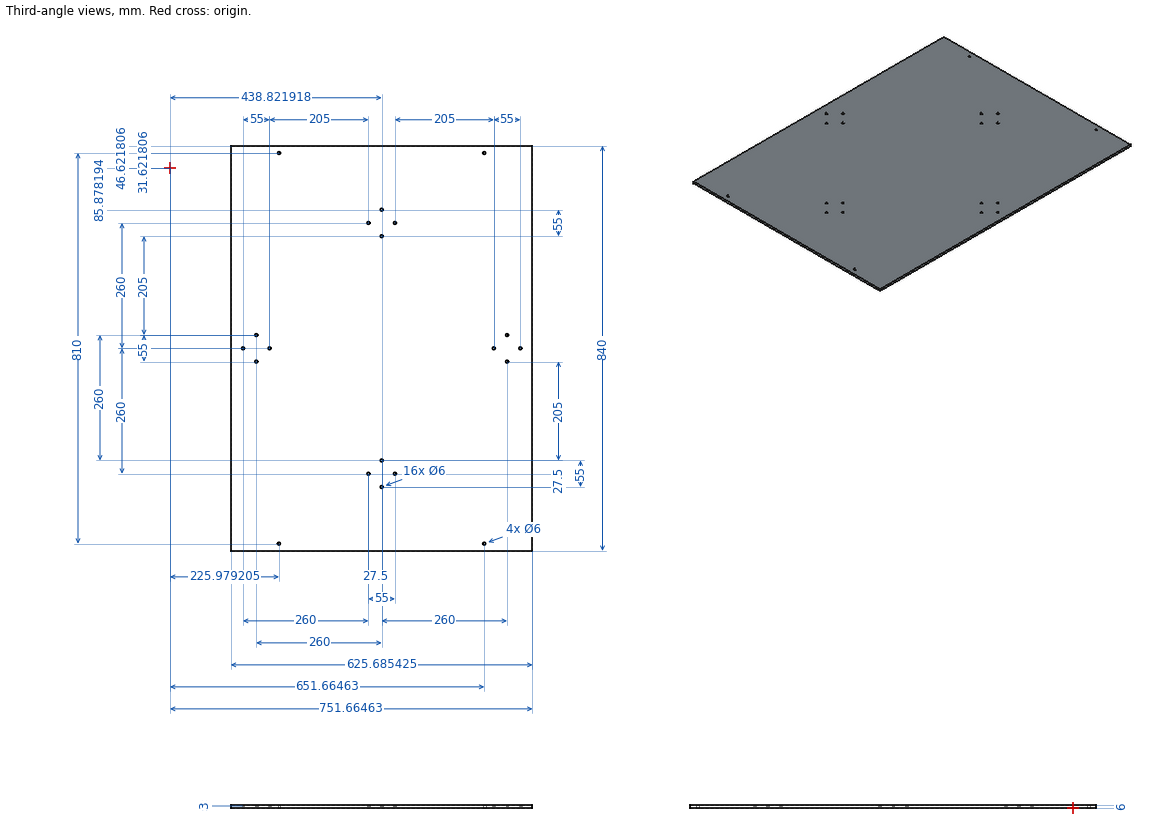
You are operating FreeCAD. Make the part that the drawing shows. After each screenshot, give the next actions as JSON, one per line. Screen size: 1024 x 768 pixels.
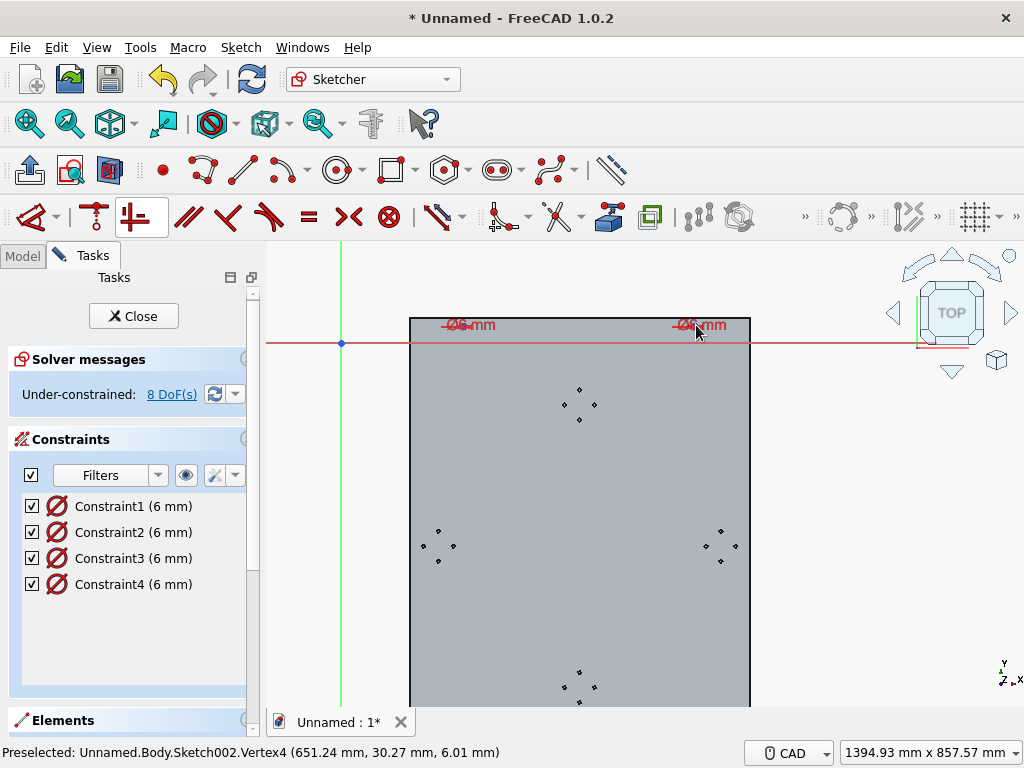
{"action": "scroll", "coordinate": [693, 327], "scroll_direction": "down", "scroll_amount": 2}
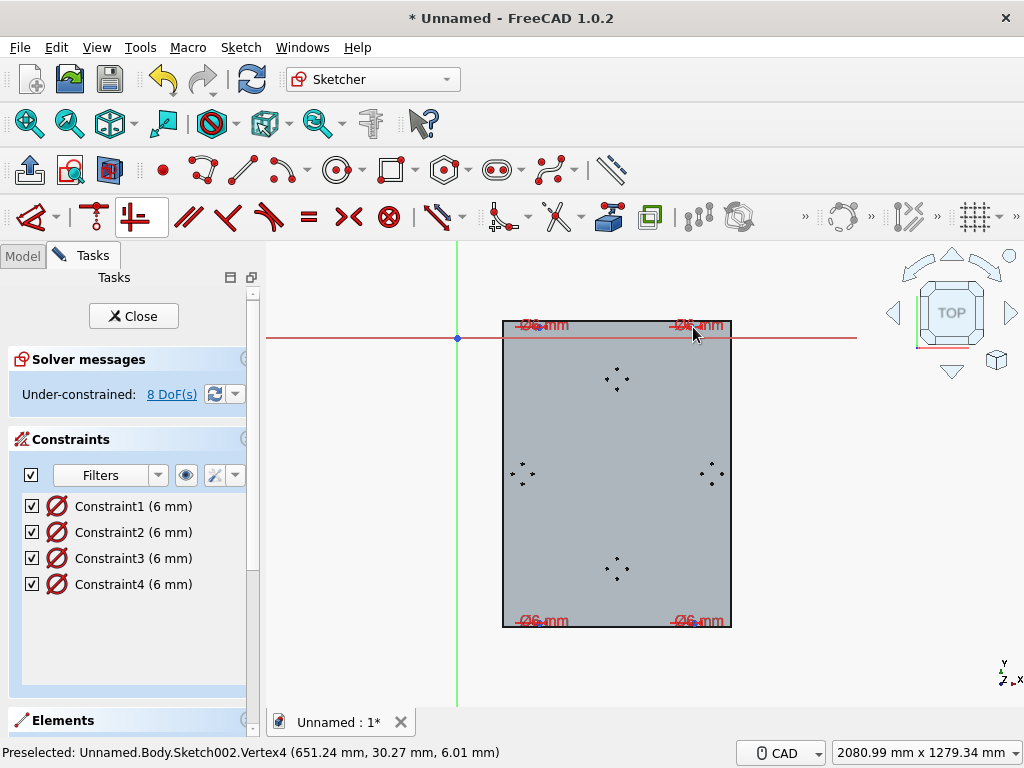
{"action": "left_click", "coordinate": [695, 623]}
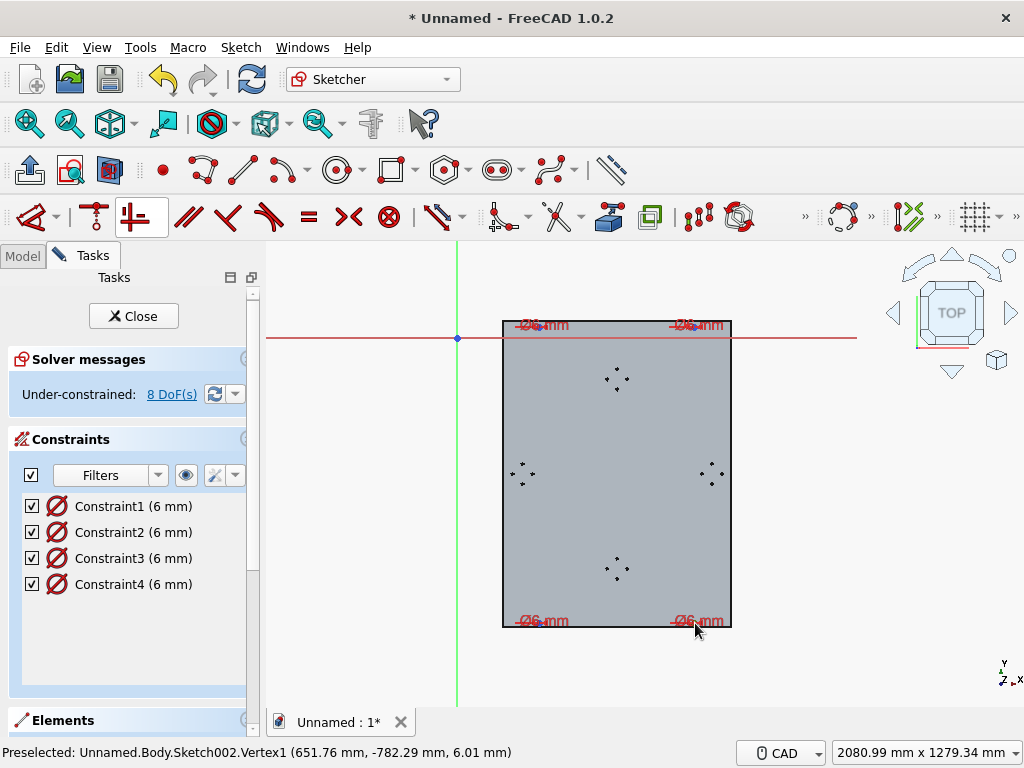
{"action": "left_click", "coordinate": [540, 623]}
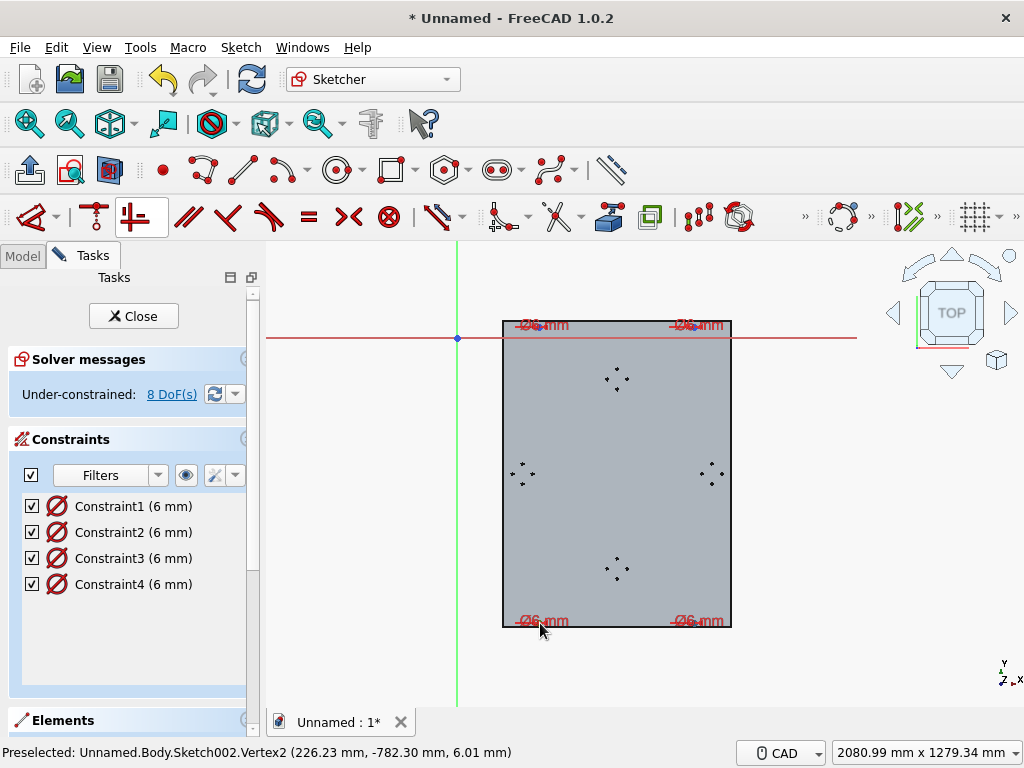
{"action": "left_click", "coordinate": [162, 218]}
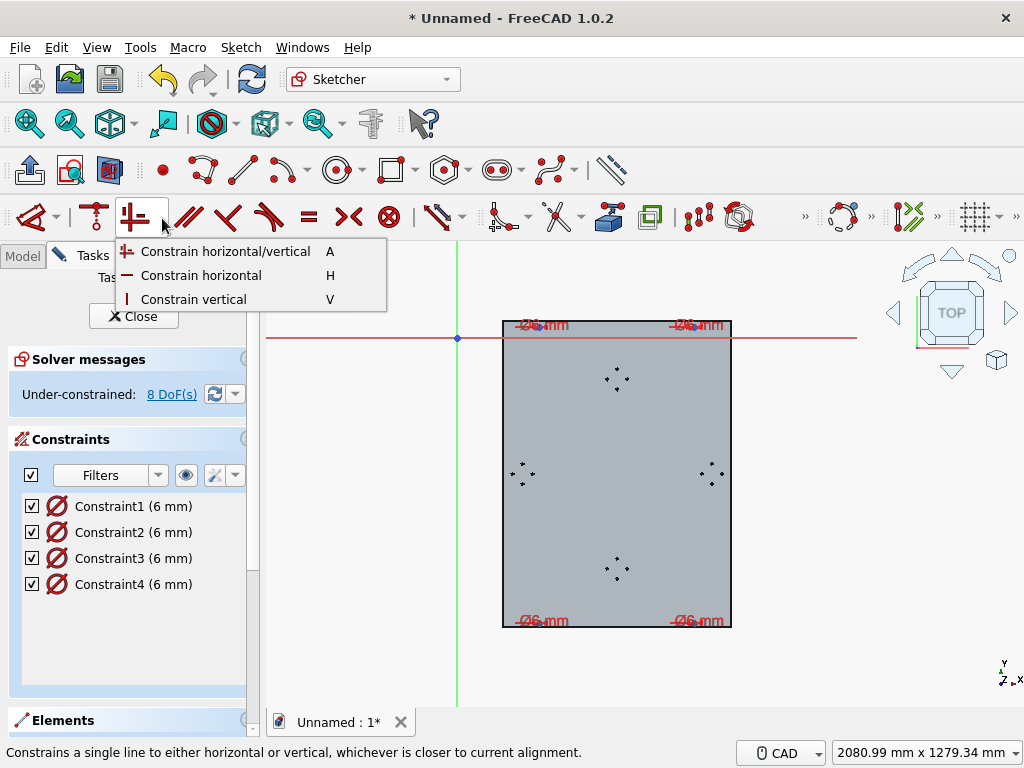
{"action": "left_click", "coordinate": [251, 275]}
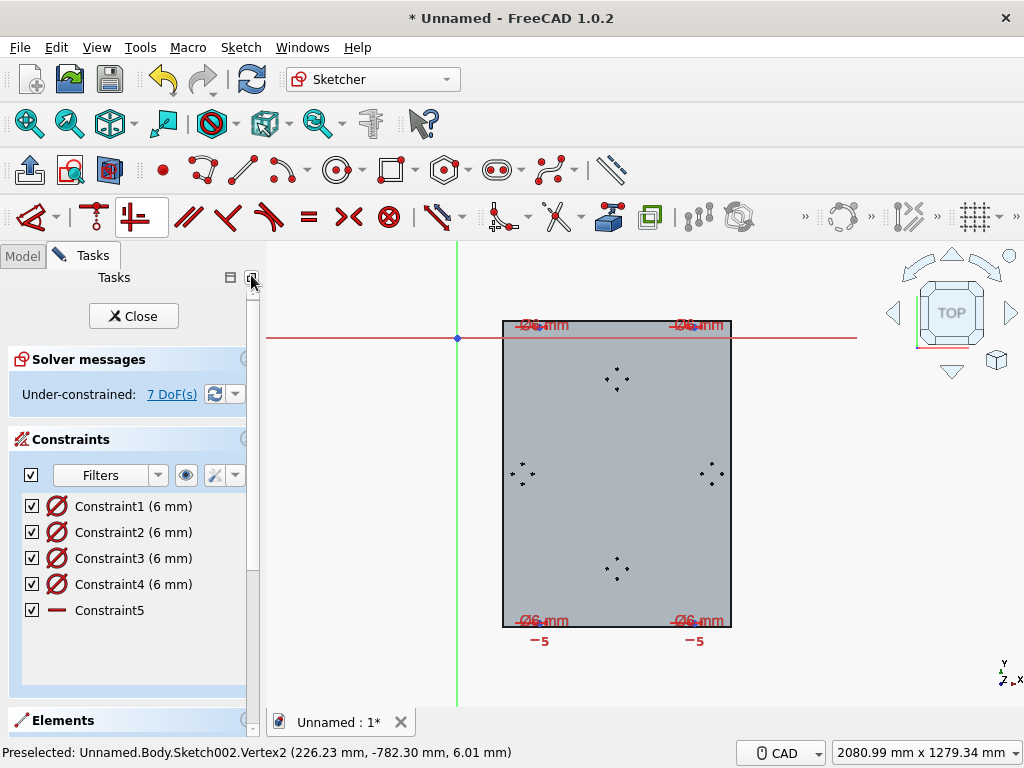
{"action": "left_click", "coordinate": [540, 623]}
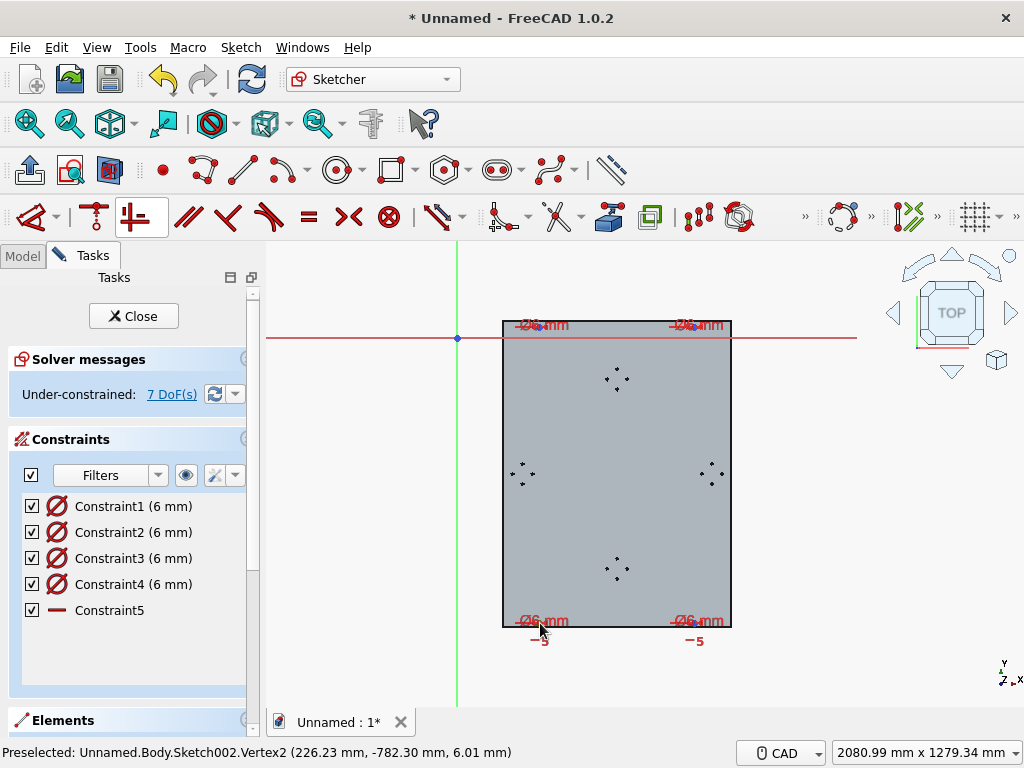
{"action": "left_click", "coordinate": [540, 327]}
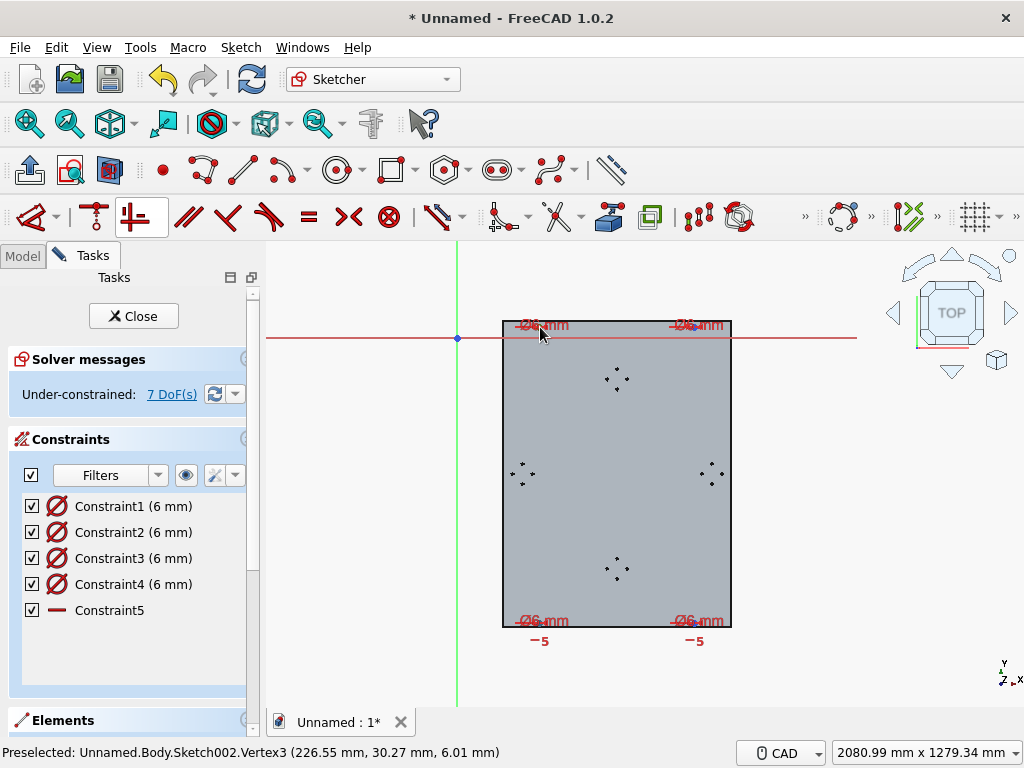
{"action": "left_click", "coordinate": [162, 218]}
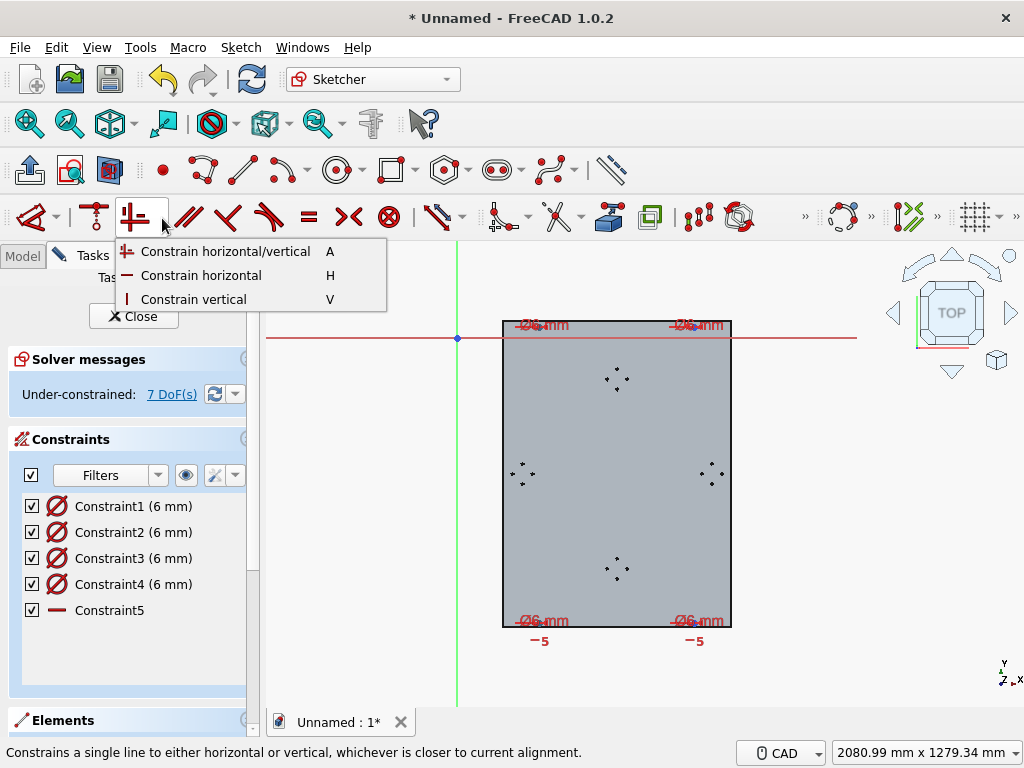
{"action": "left_click", "coordinate": [251, 299]}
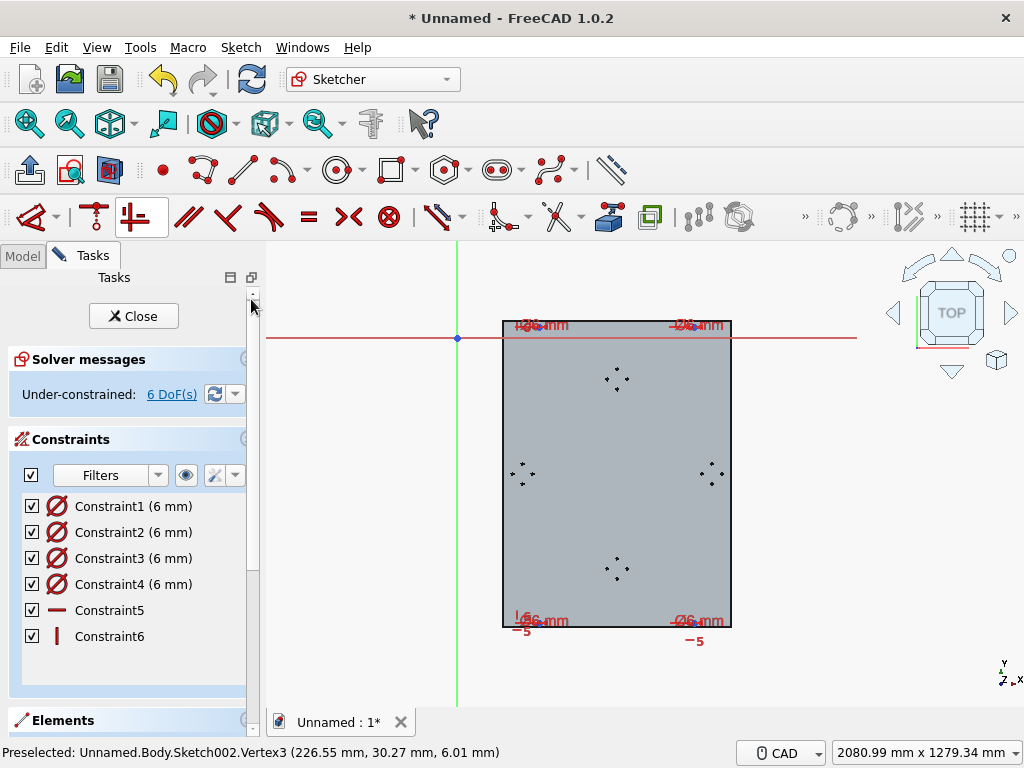
{"action": "left_click", "coordinate": [695, 623]}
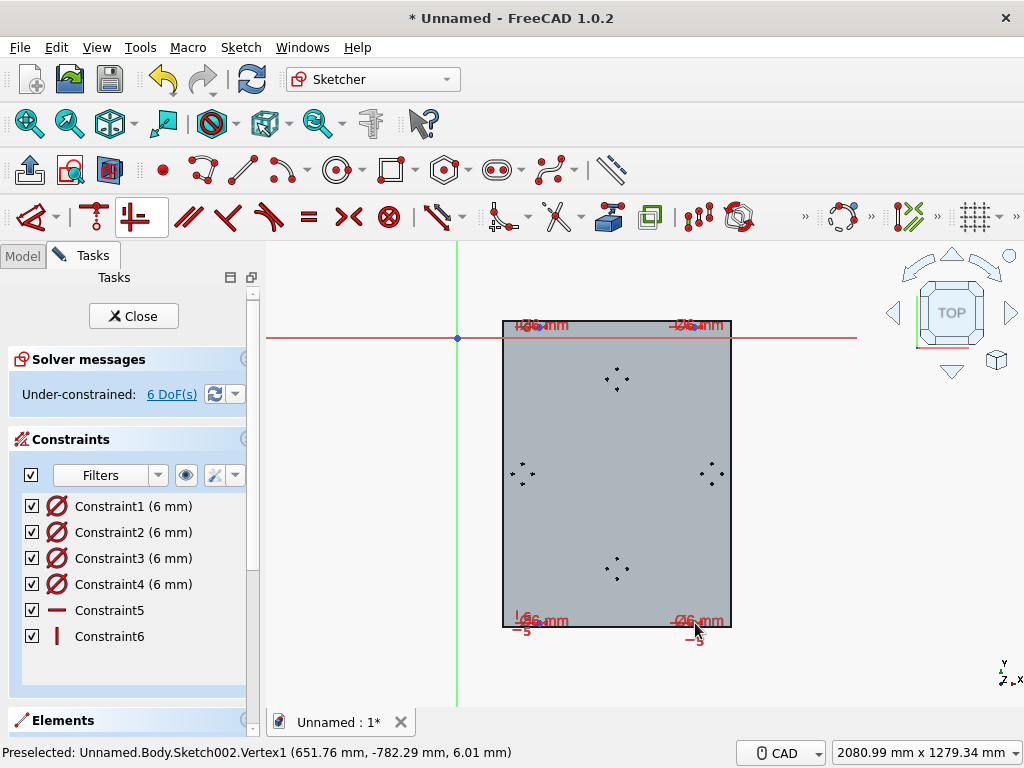
{"action": "left_click", "coordinate": [695, 327]}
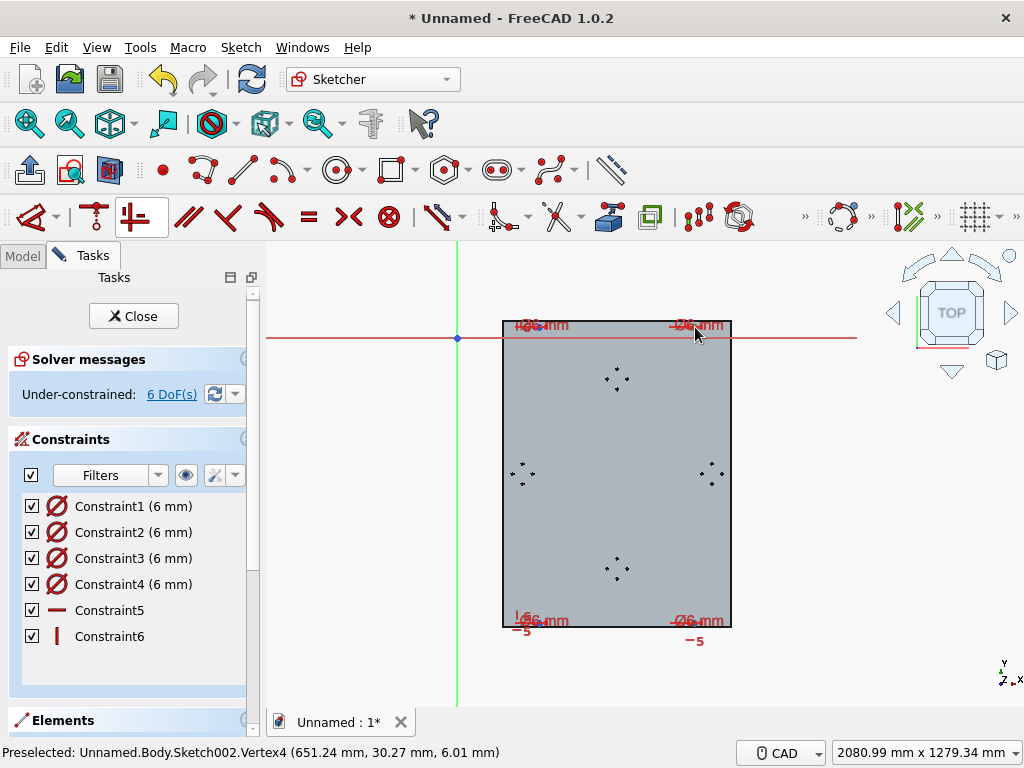
{"action": "left_click", "coordinate": [162, 218]}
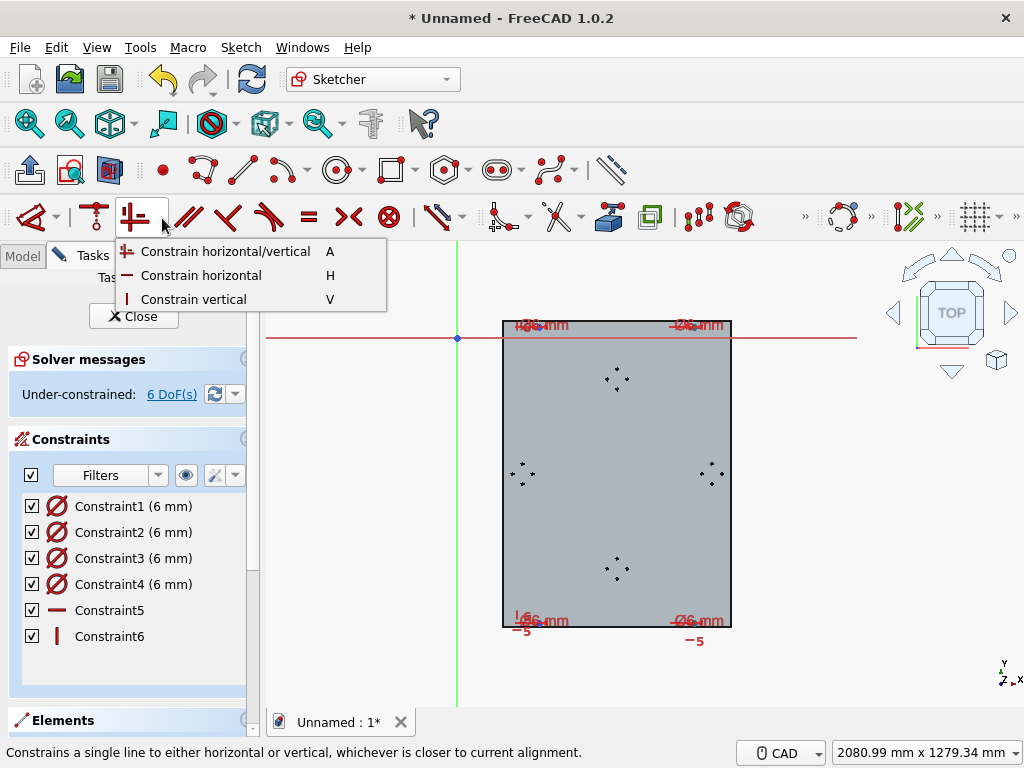
{"action": "left_click", "coordinate": [251, 299]}